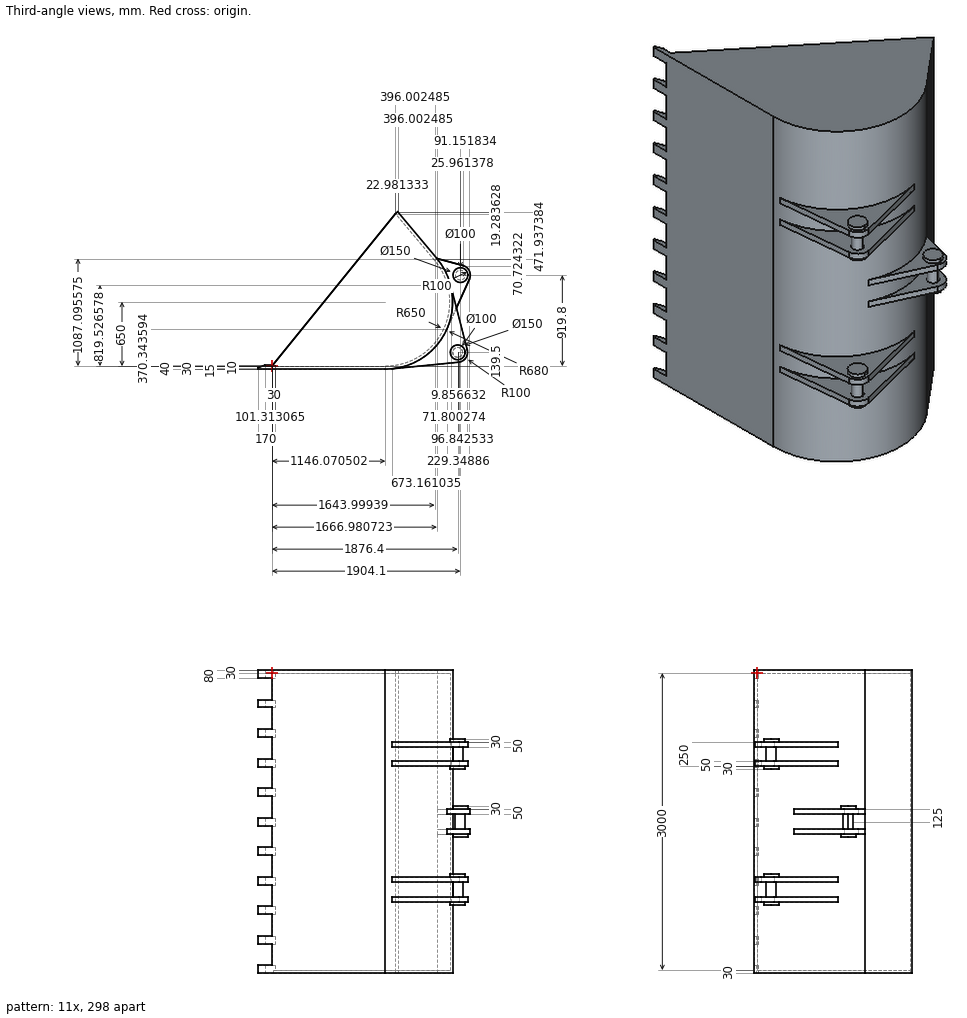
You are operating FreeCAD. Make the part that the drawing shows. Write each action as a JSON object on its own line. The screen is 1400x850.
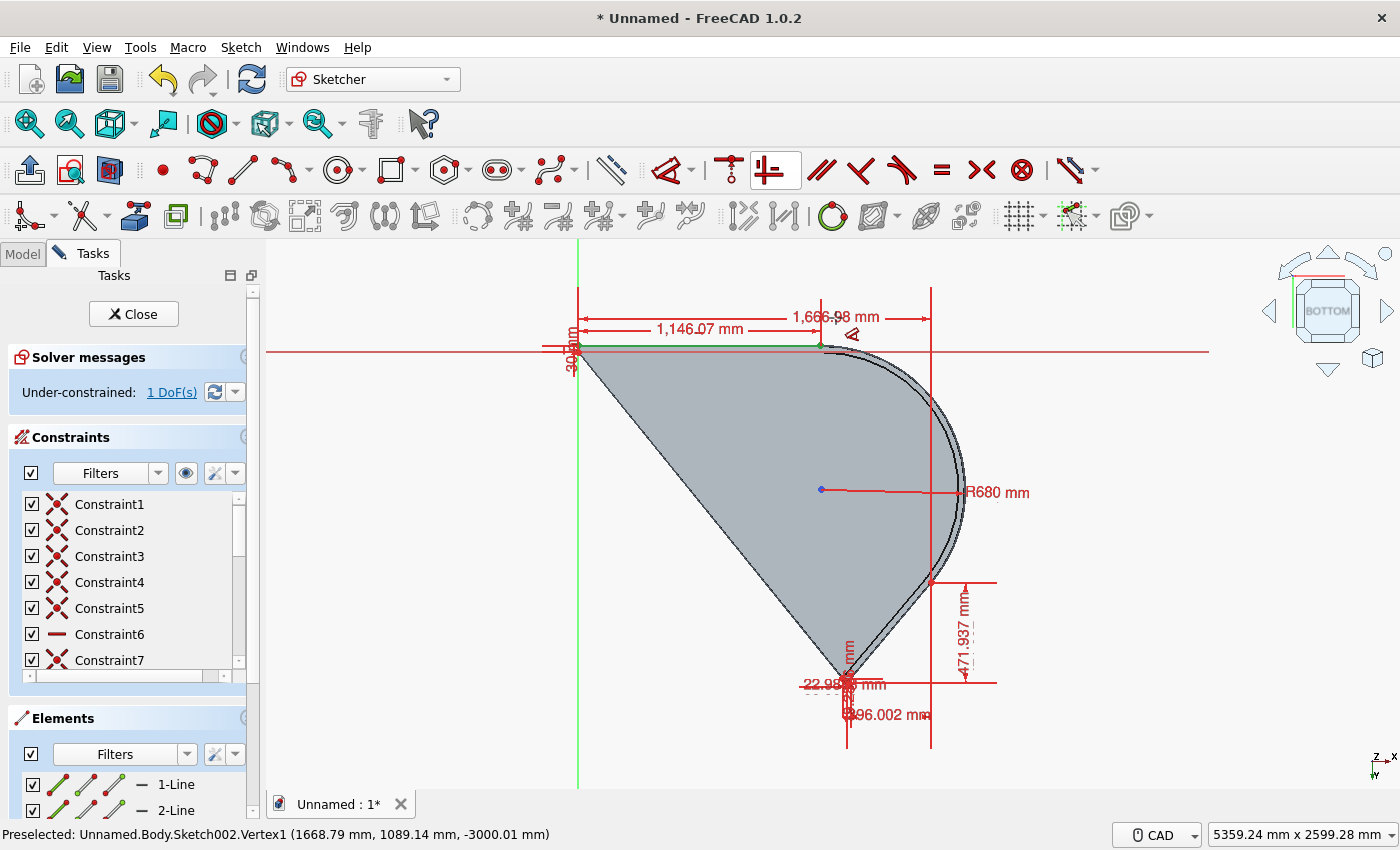
{"action": "left_click", "coordinate": [931, 583]}
{"action": "left_click", "coordinate": [544, 467]}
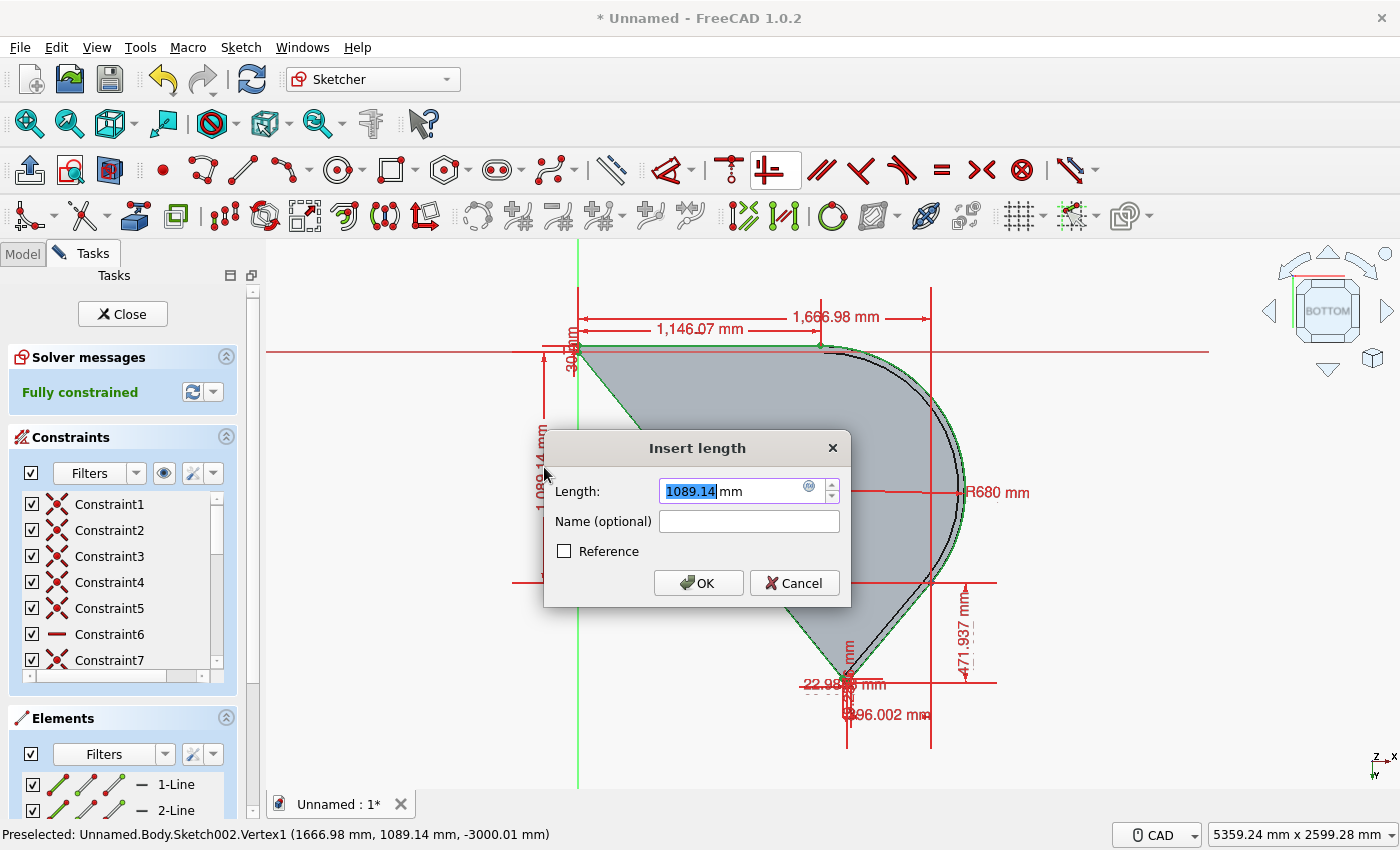
{"action": "type", "text": "1087.095575"}
{"action": "key", "text": "Return"}
{"action": "key", "text": "Escape"}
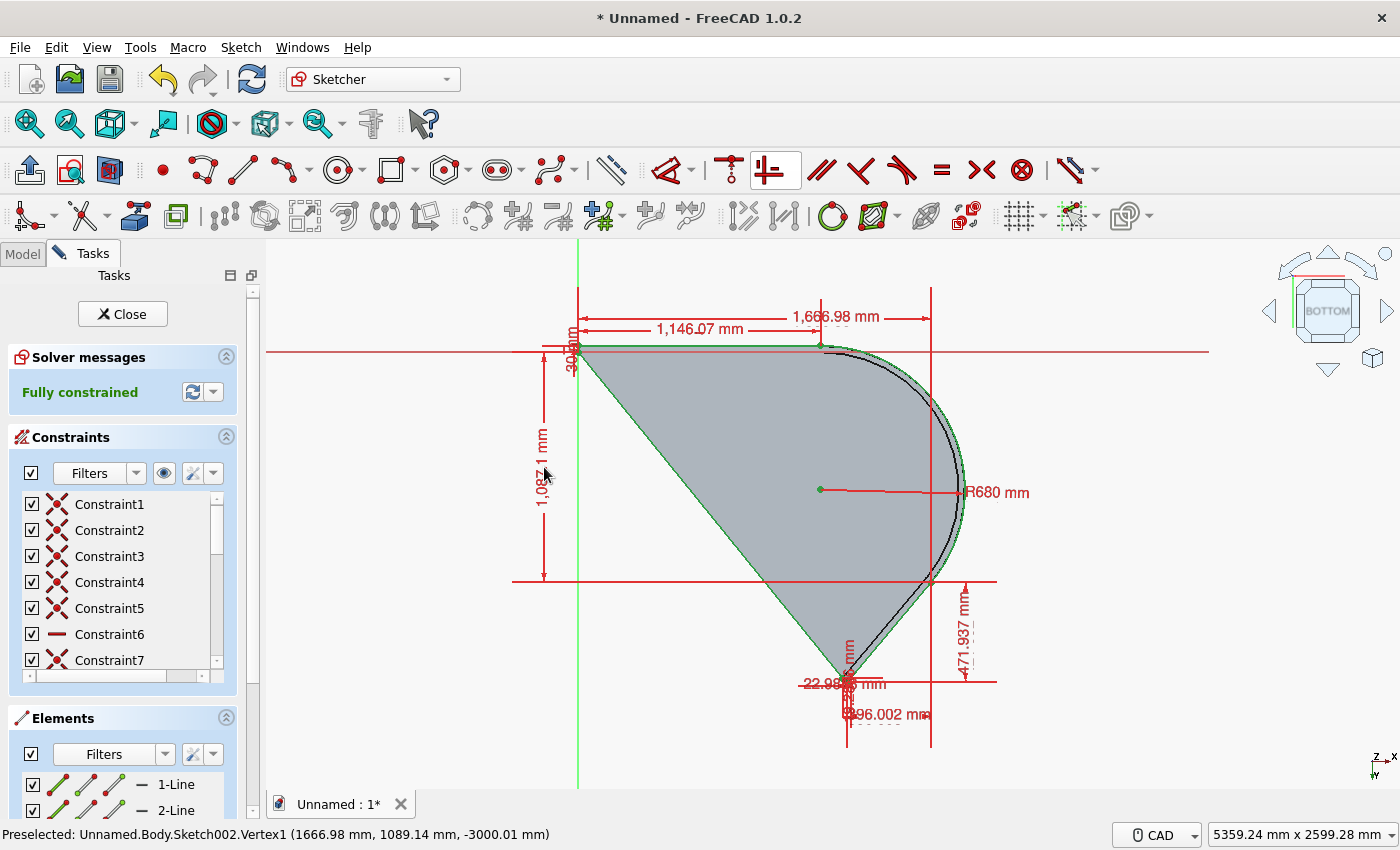
{"action": "left_click", "coordinate": [123, 314]}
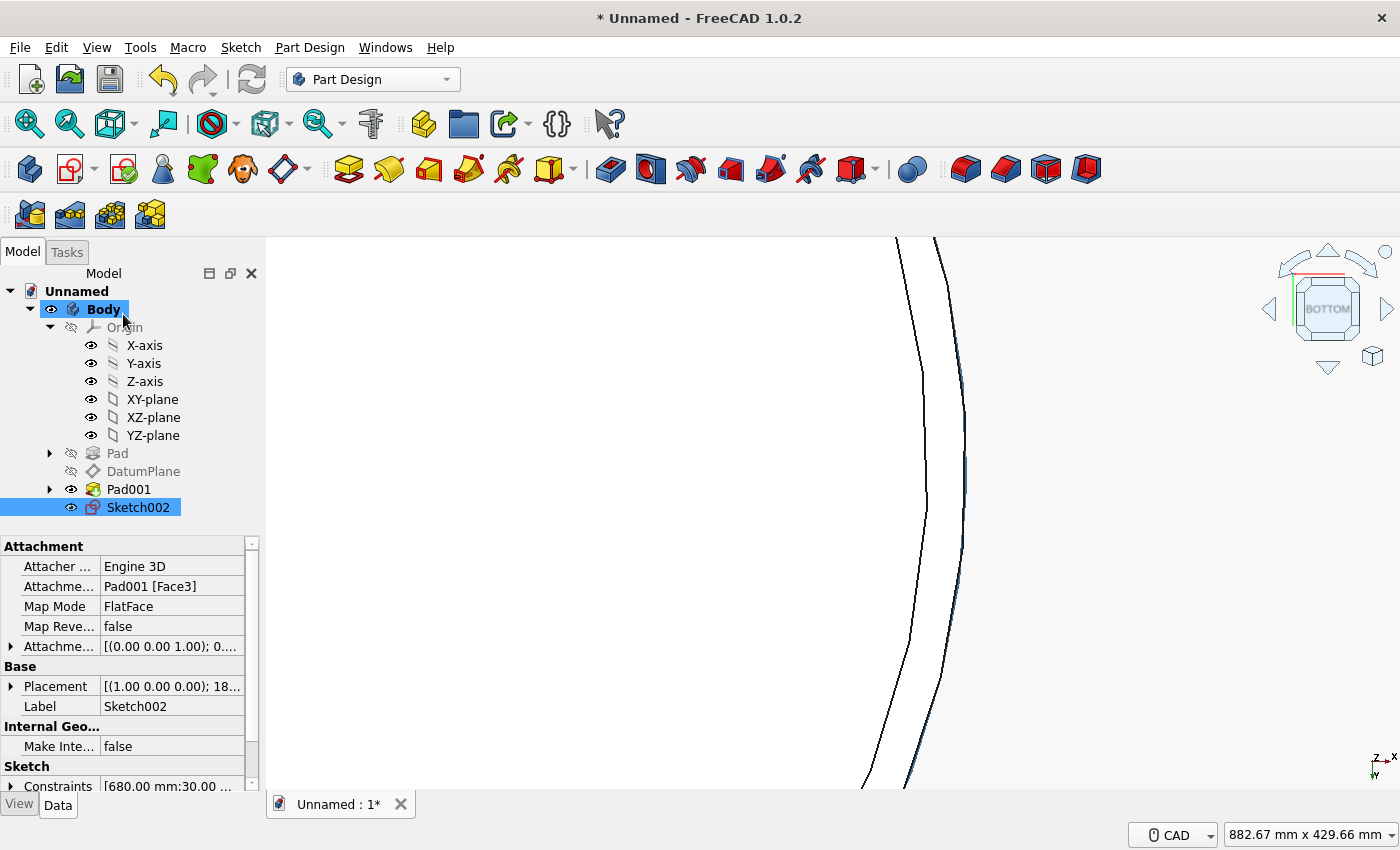
{"action": "left_click", "coordinate": [350, 170]}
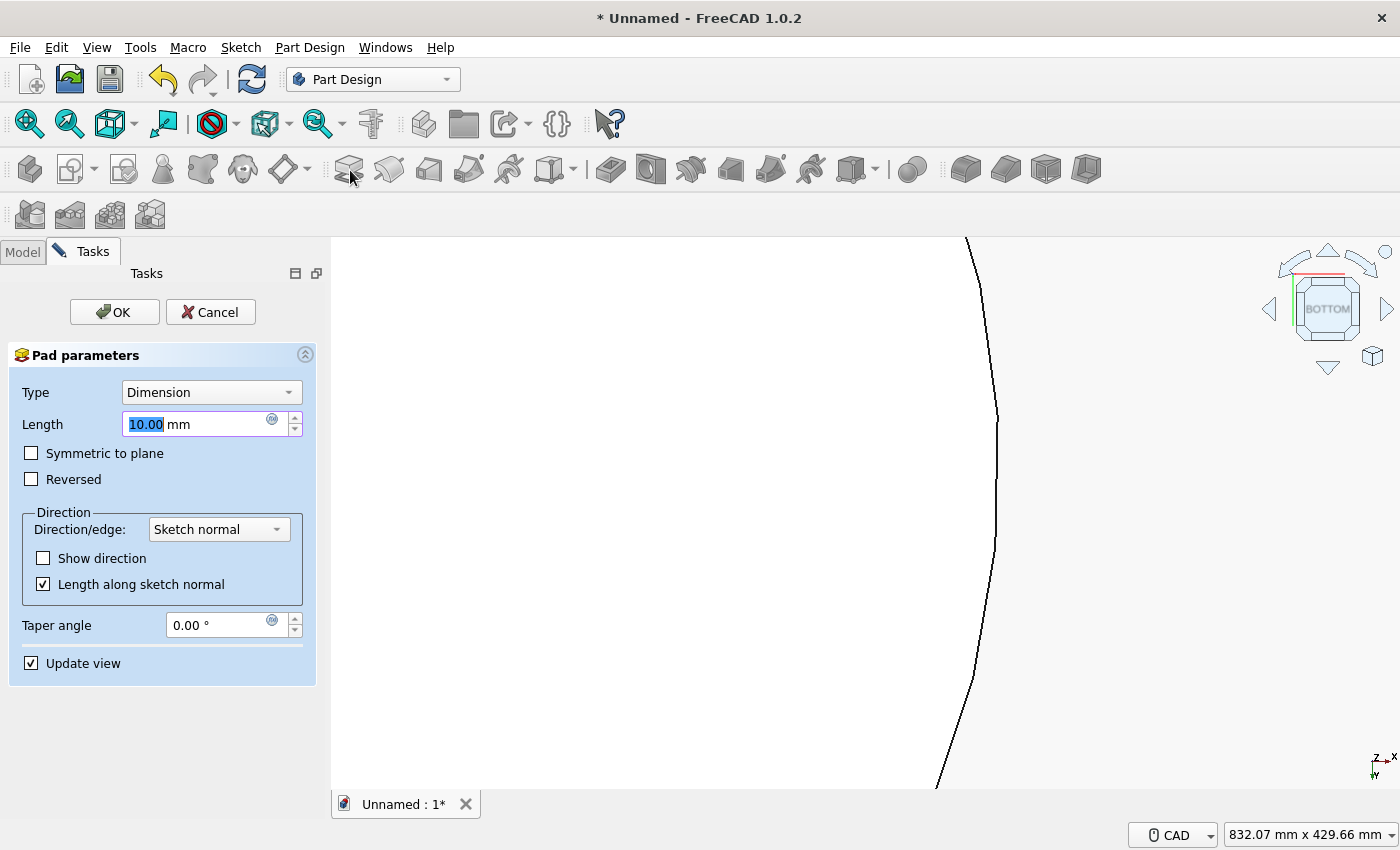
{"action": "type", "text": "30"}
{"action": "key", "text": "Tab"}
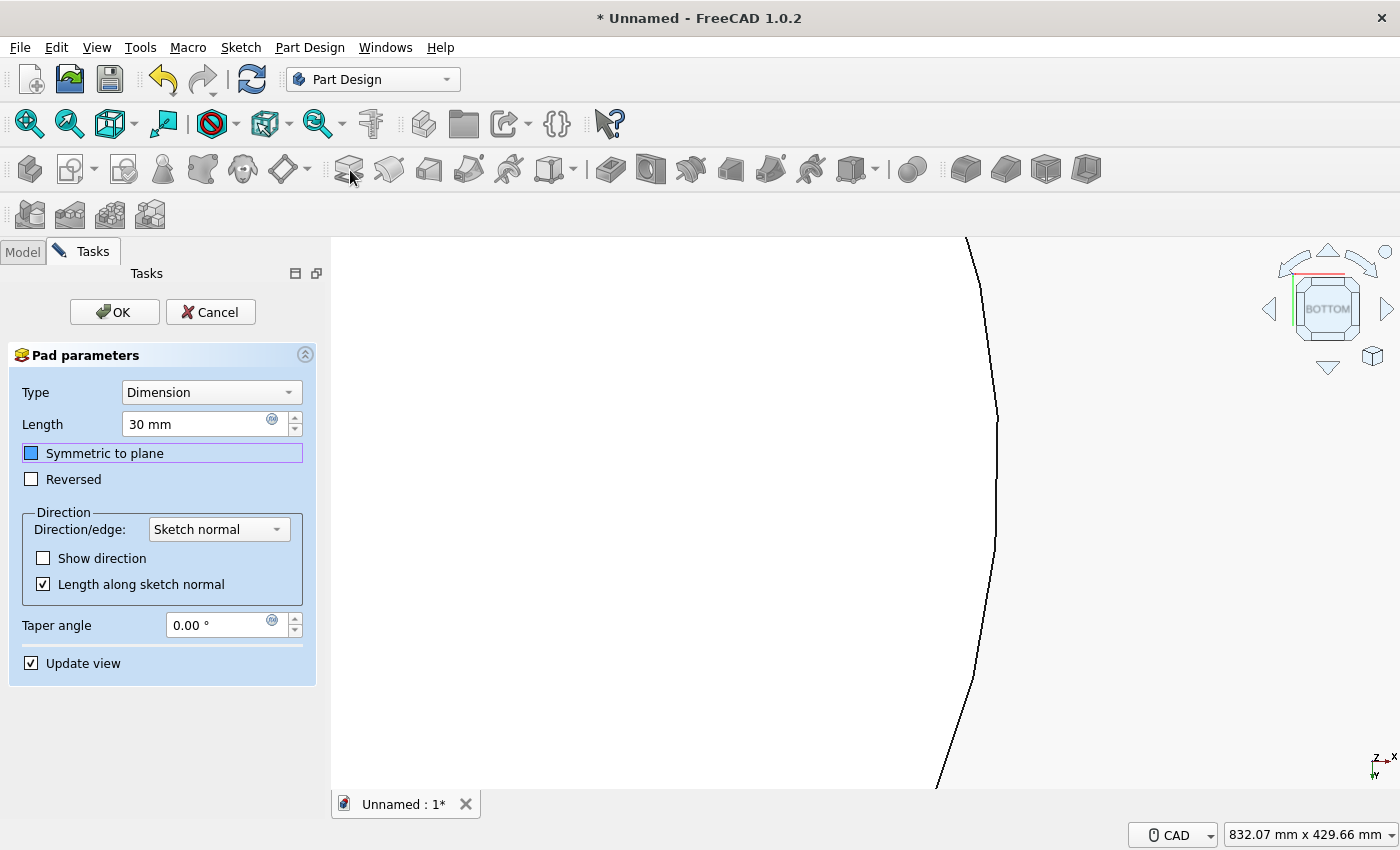
{"action": "left_click", "coordinate": [115, 312]}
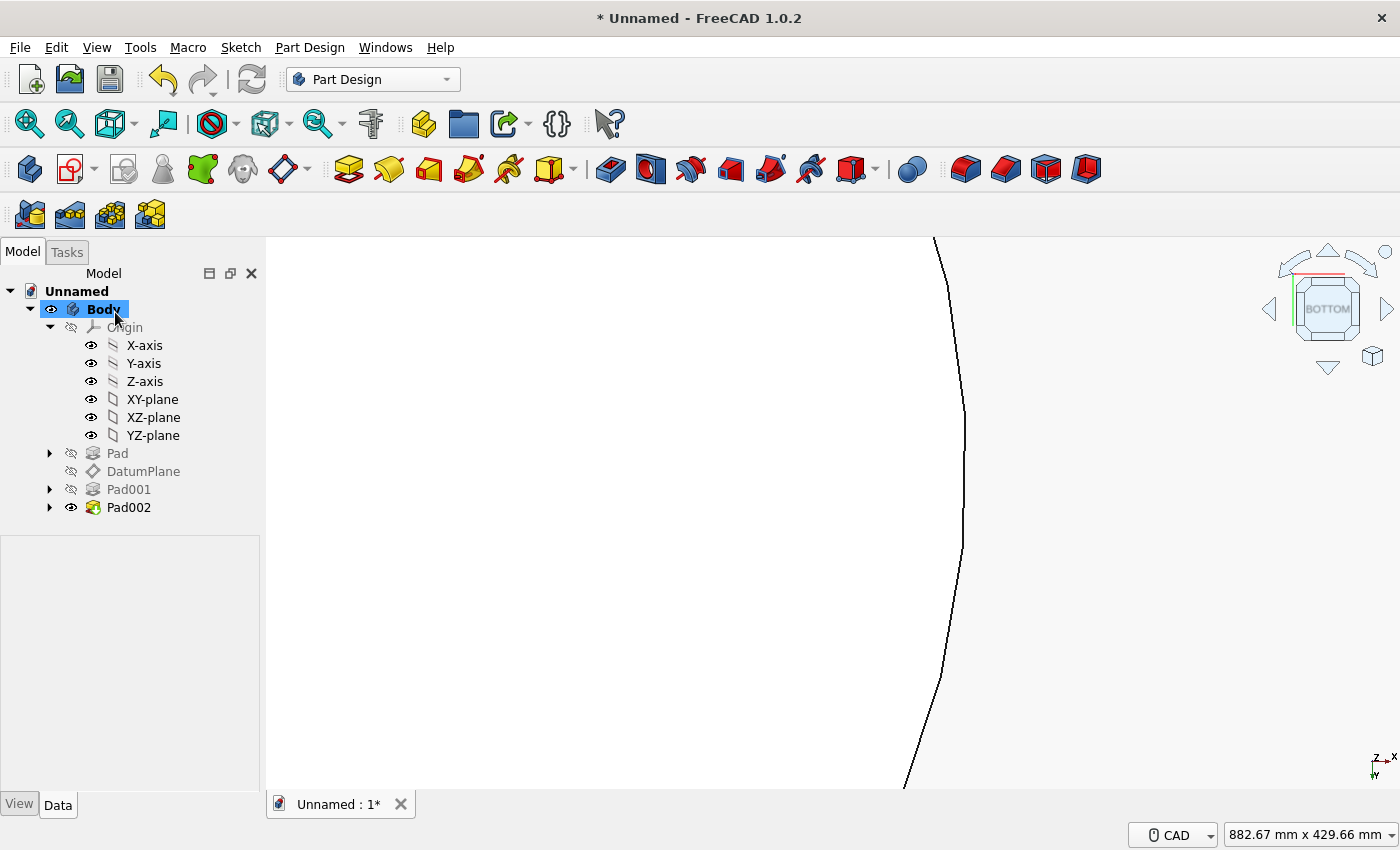
{"action": "key", "text": "v f"}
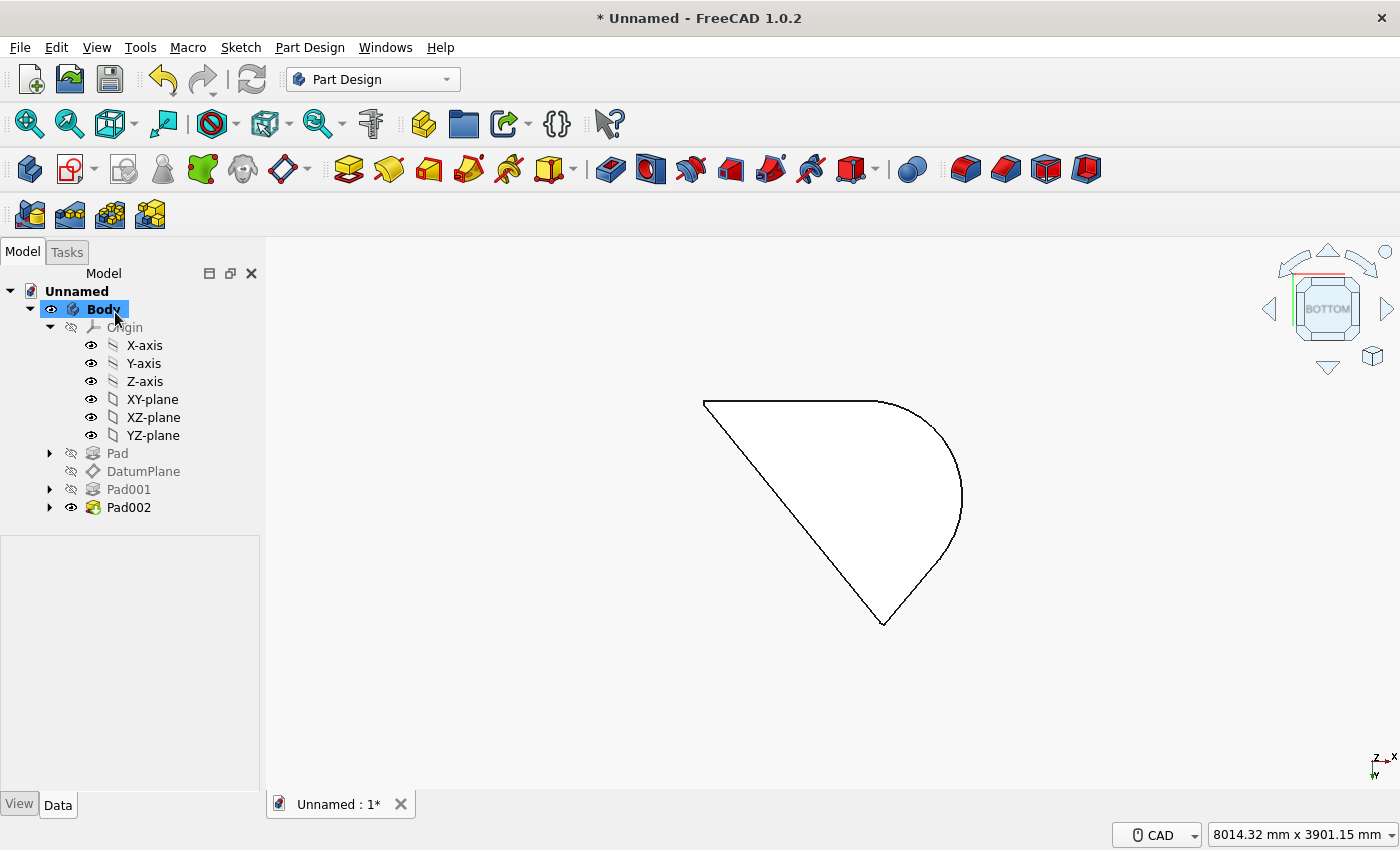
{"action": "left_click", "coordinate": [136, 399]}